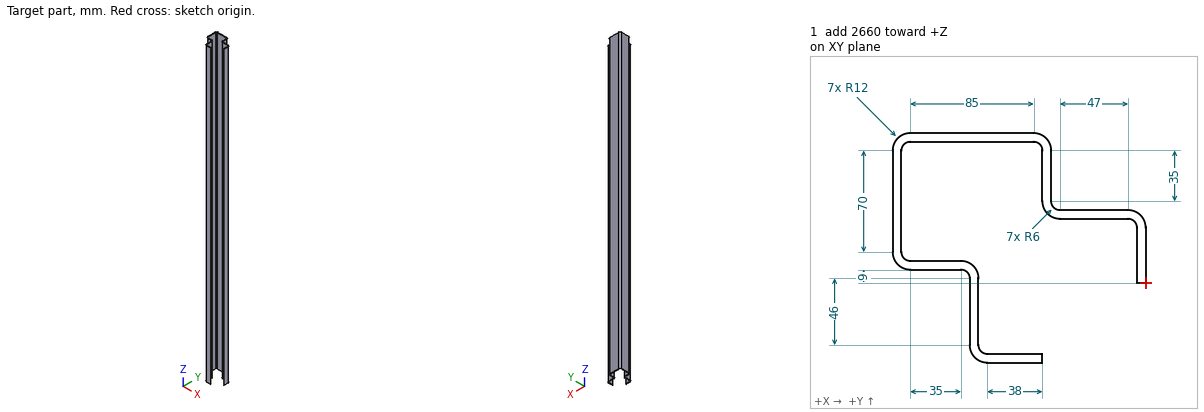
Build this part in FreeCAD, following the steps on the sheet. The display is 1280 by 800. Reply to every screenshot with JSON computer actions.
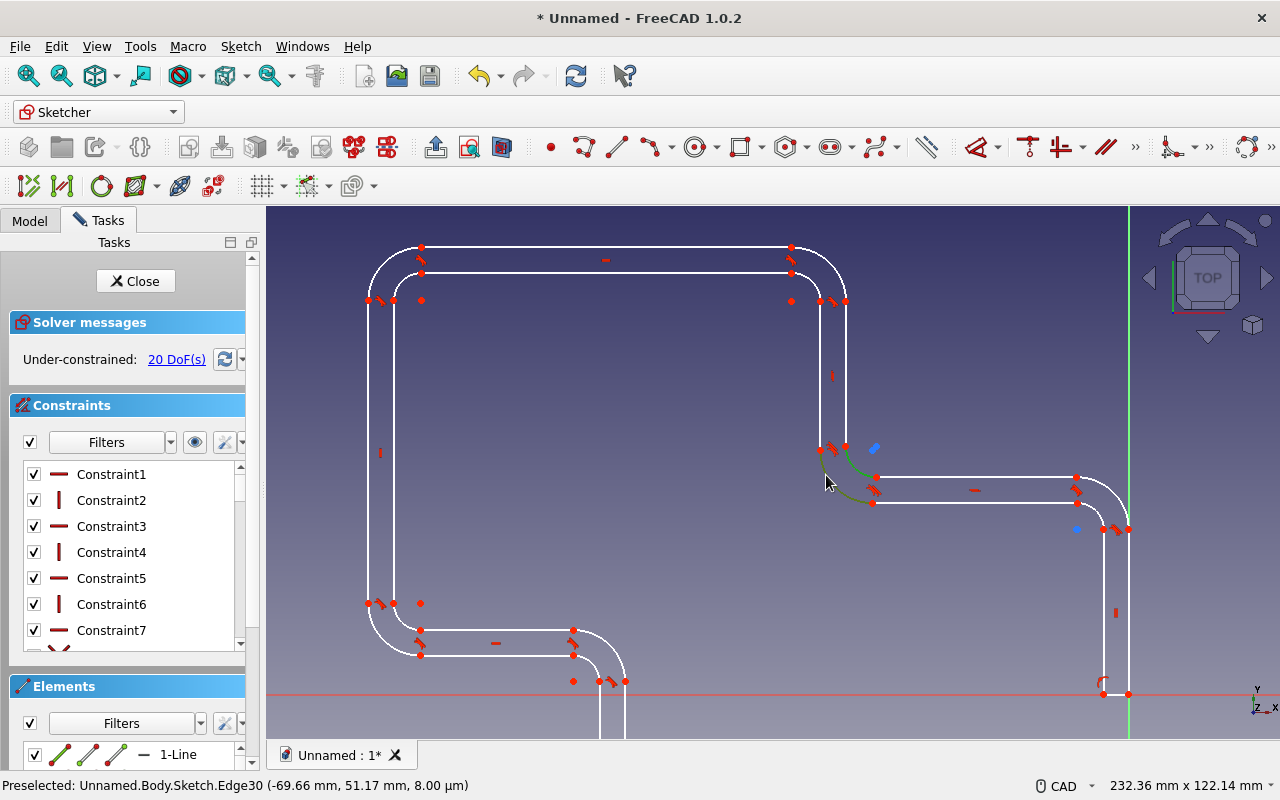
{"action": "key", "text": "c"}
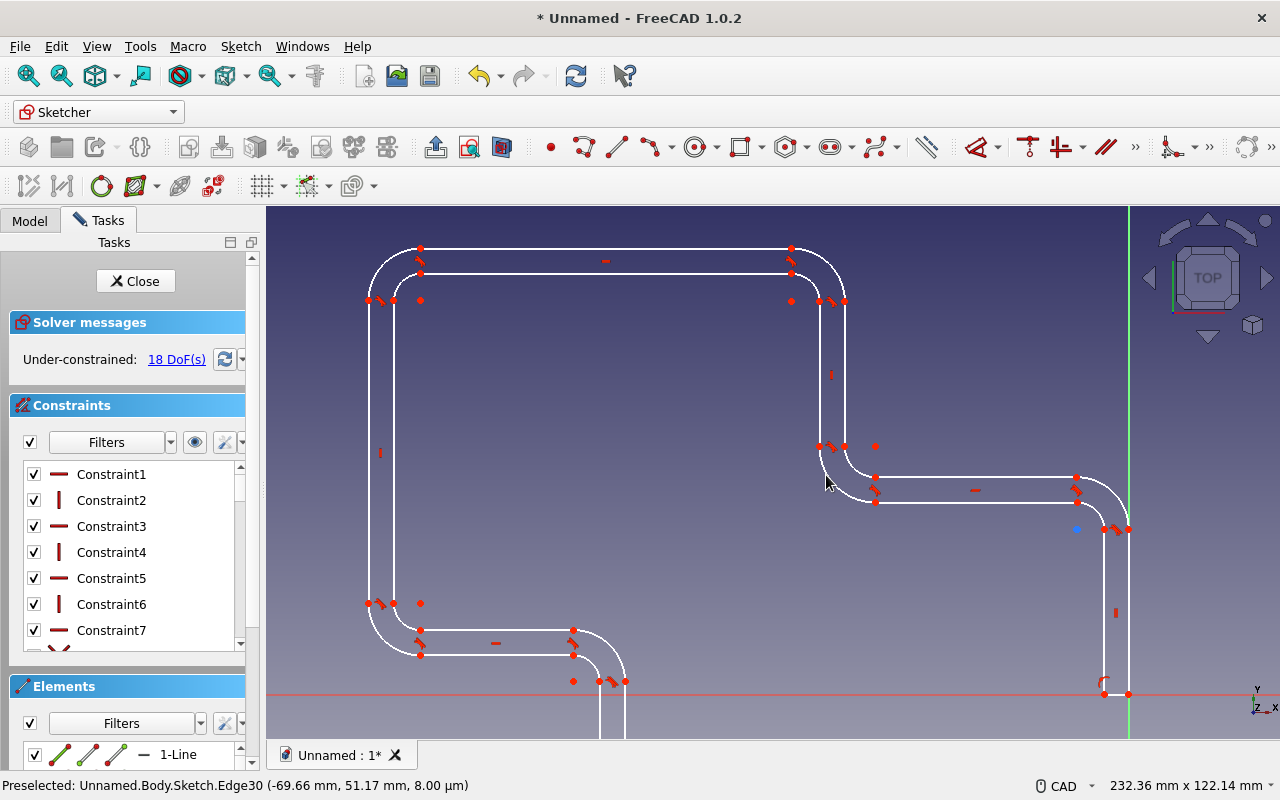
{"action": "left_click", "coordinate": [1101, 517]}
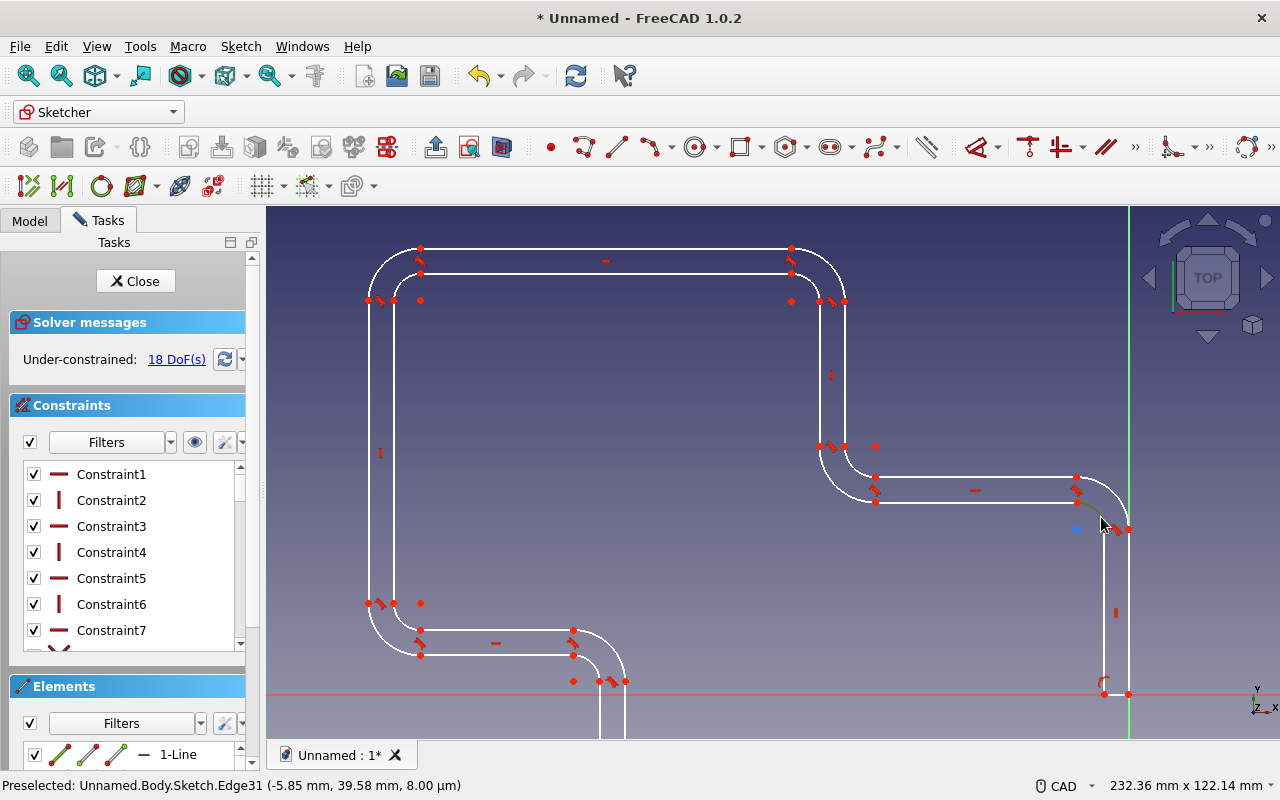
{"action": "left_click", "coordinate": [1100, 483]}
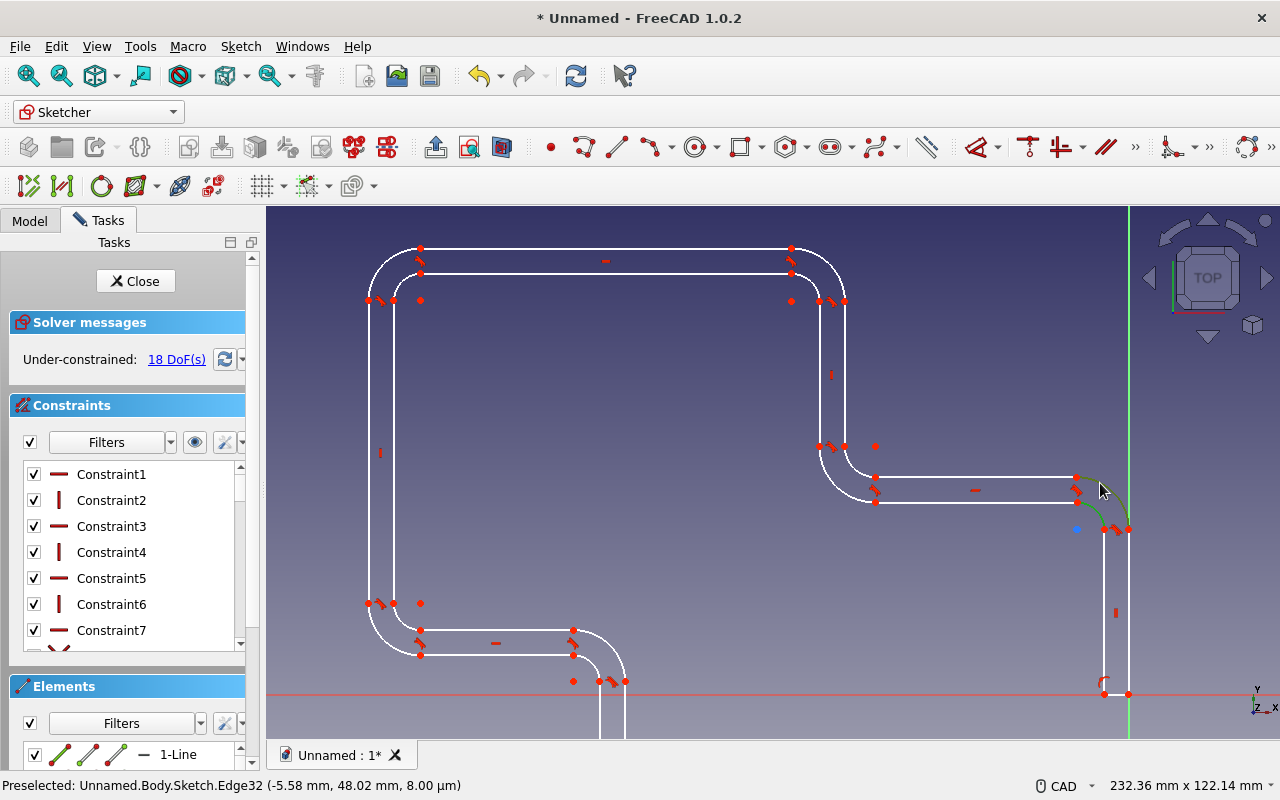
{"action": "left_click", "coordinate": [1028, 148]}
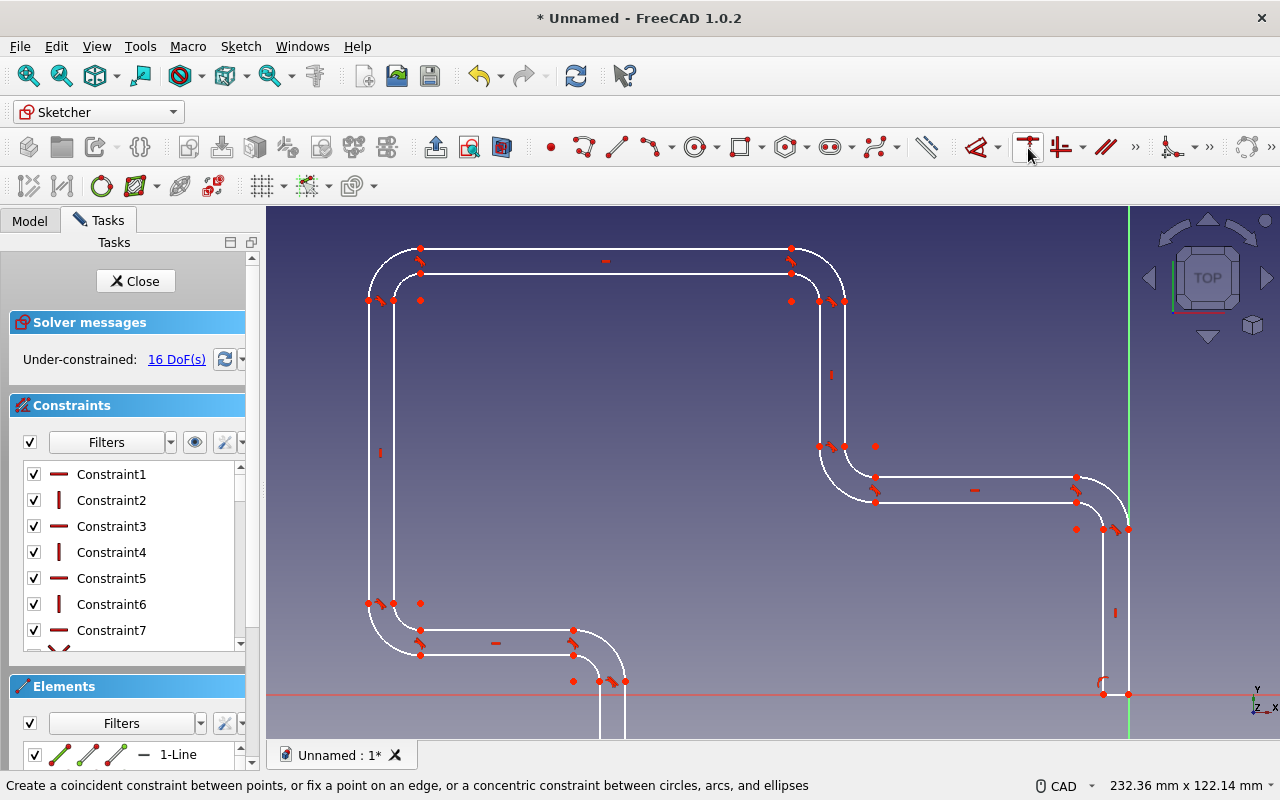
{"action": "left_click", "coordinate": [839, 278]}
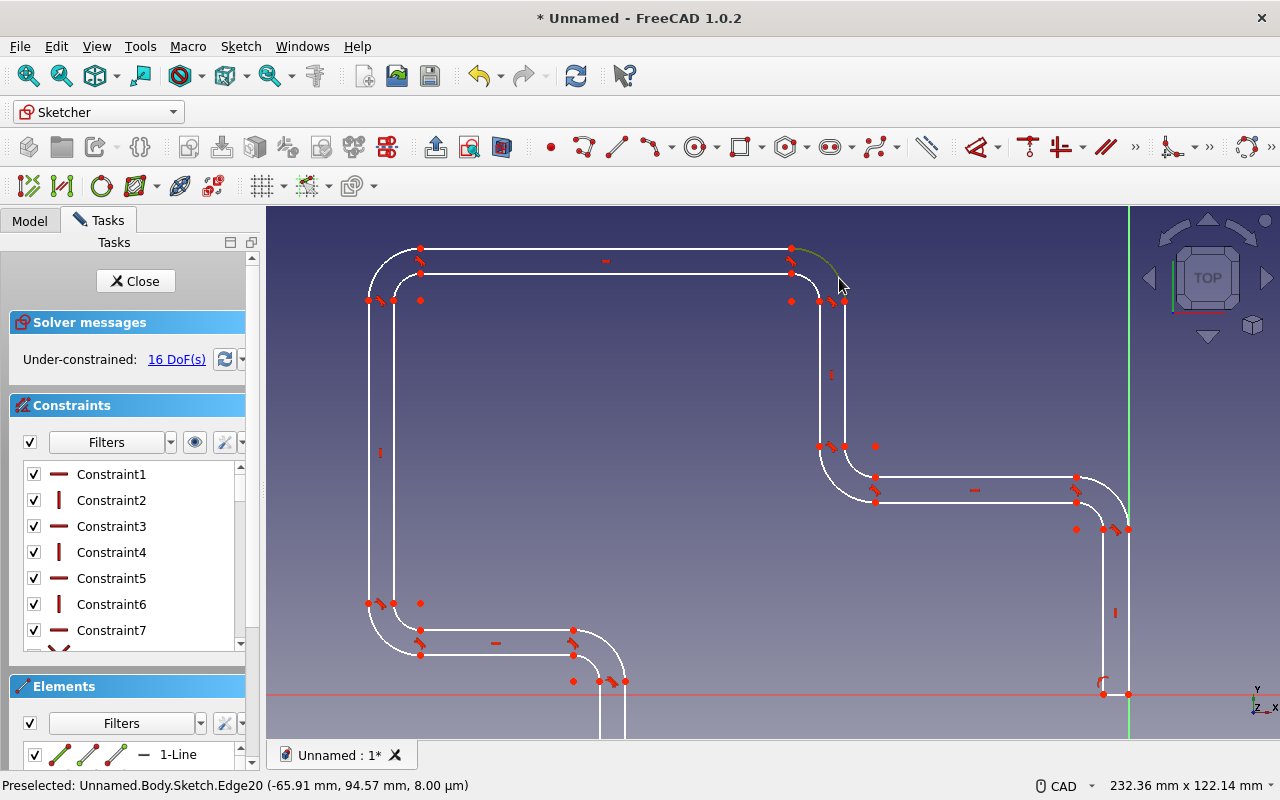
{"action": "left_click", "coordinate": [397, 254]}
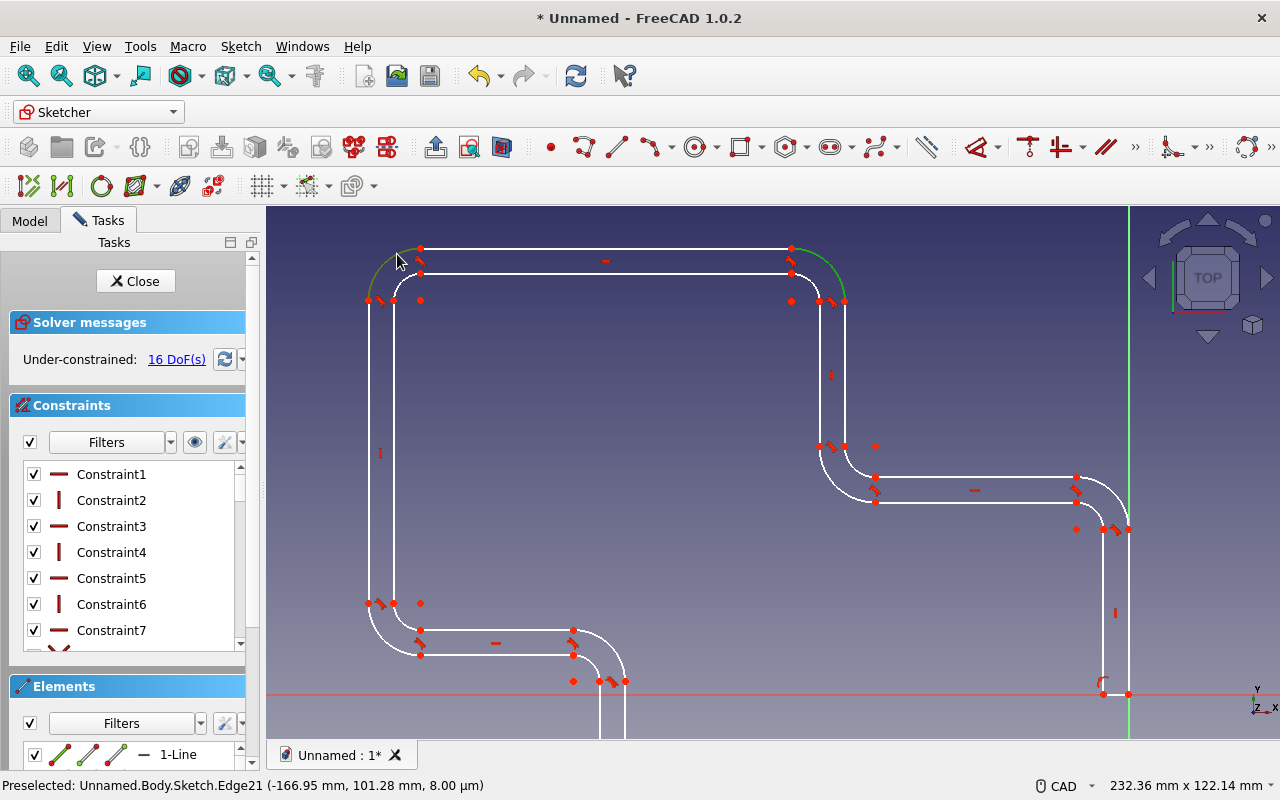
{"action": "left_click", "coordinate": [374, 627]}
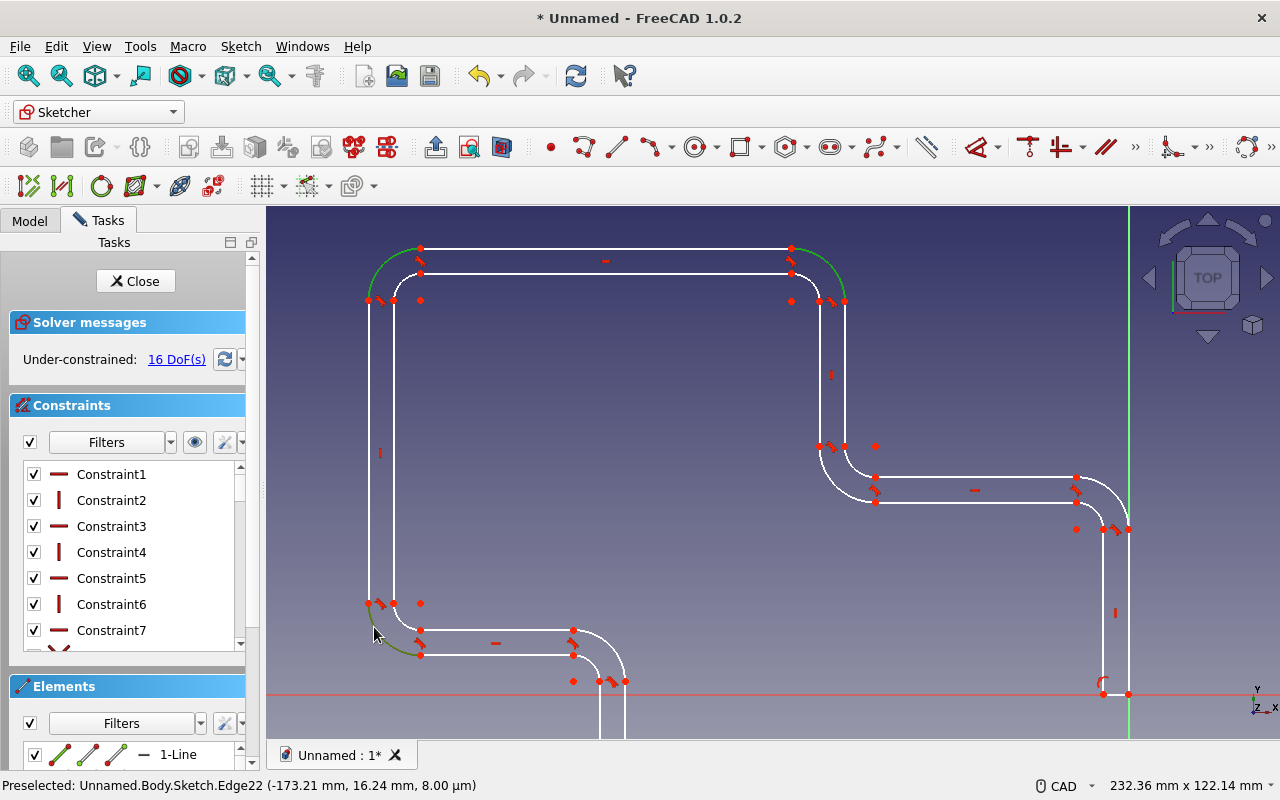
{"action": "scroll", "coordinate": [668, 377], "scroll_direction": "down", "scroll_amount": 4}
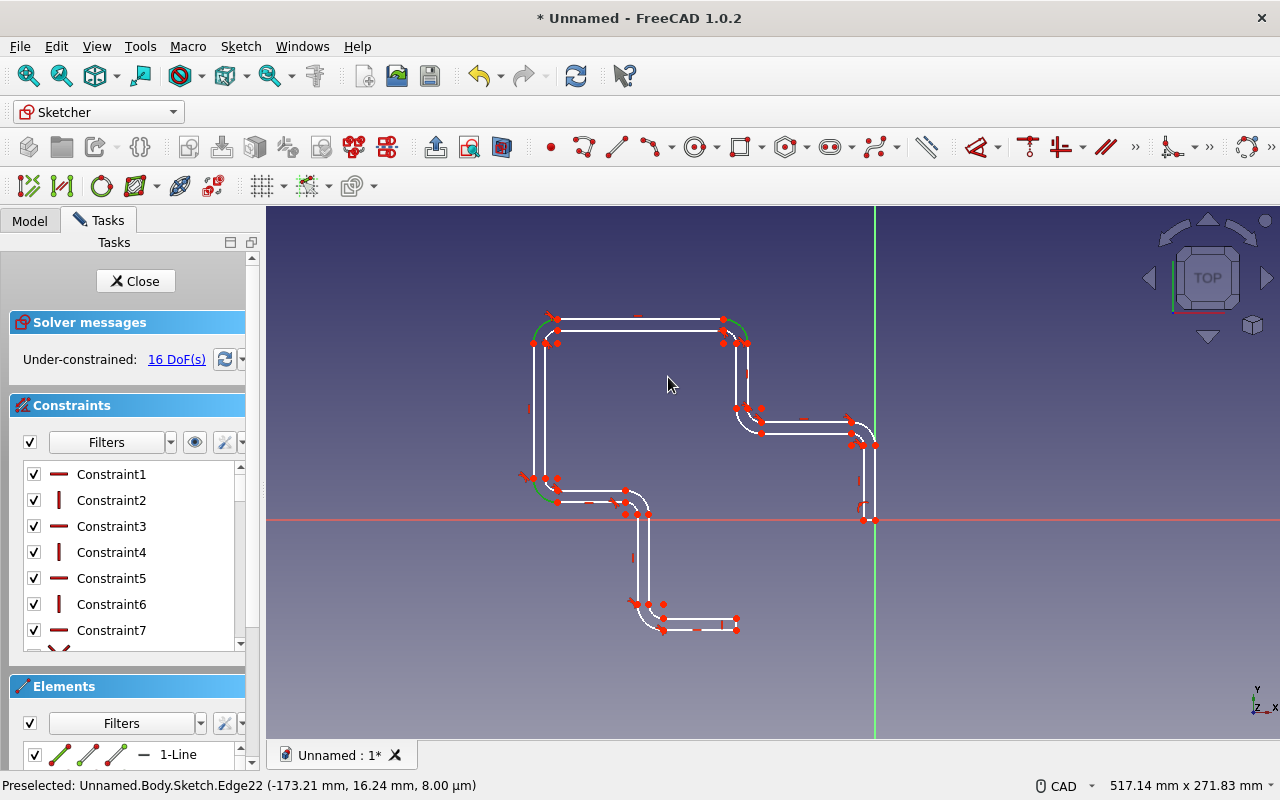
{"action": "left_click", "coordinate": [640, 616]}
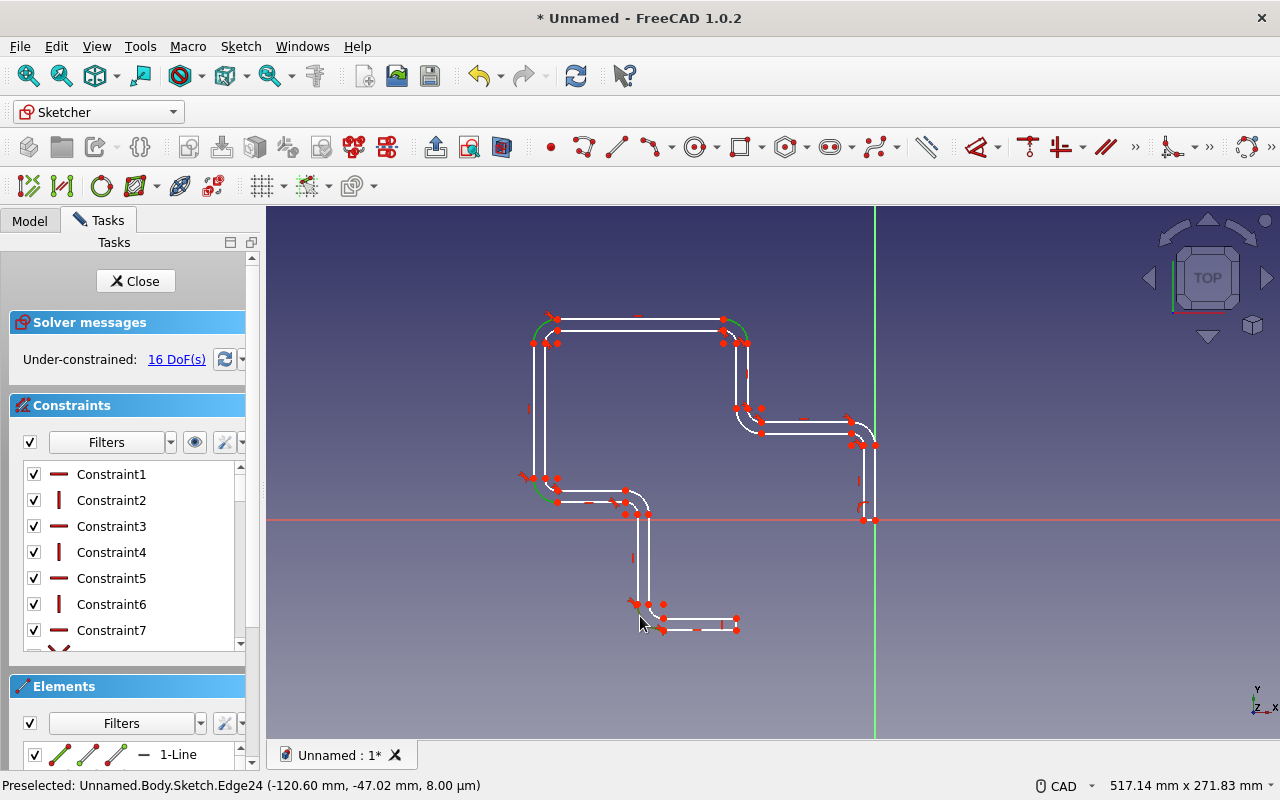
{"action": "scroll", "coordinate": [646, 504], "scroll_direction": "up", "scroll_amount": 2}